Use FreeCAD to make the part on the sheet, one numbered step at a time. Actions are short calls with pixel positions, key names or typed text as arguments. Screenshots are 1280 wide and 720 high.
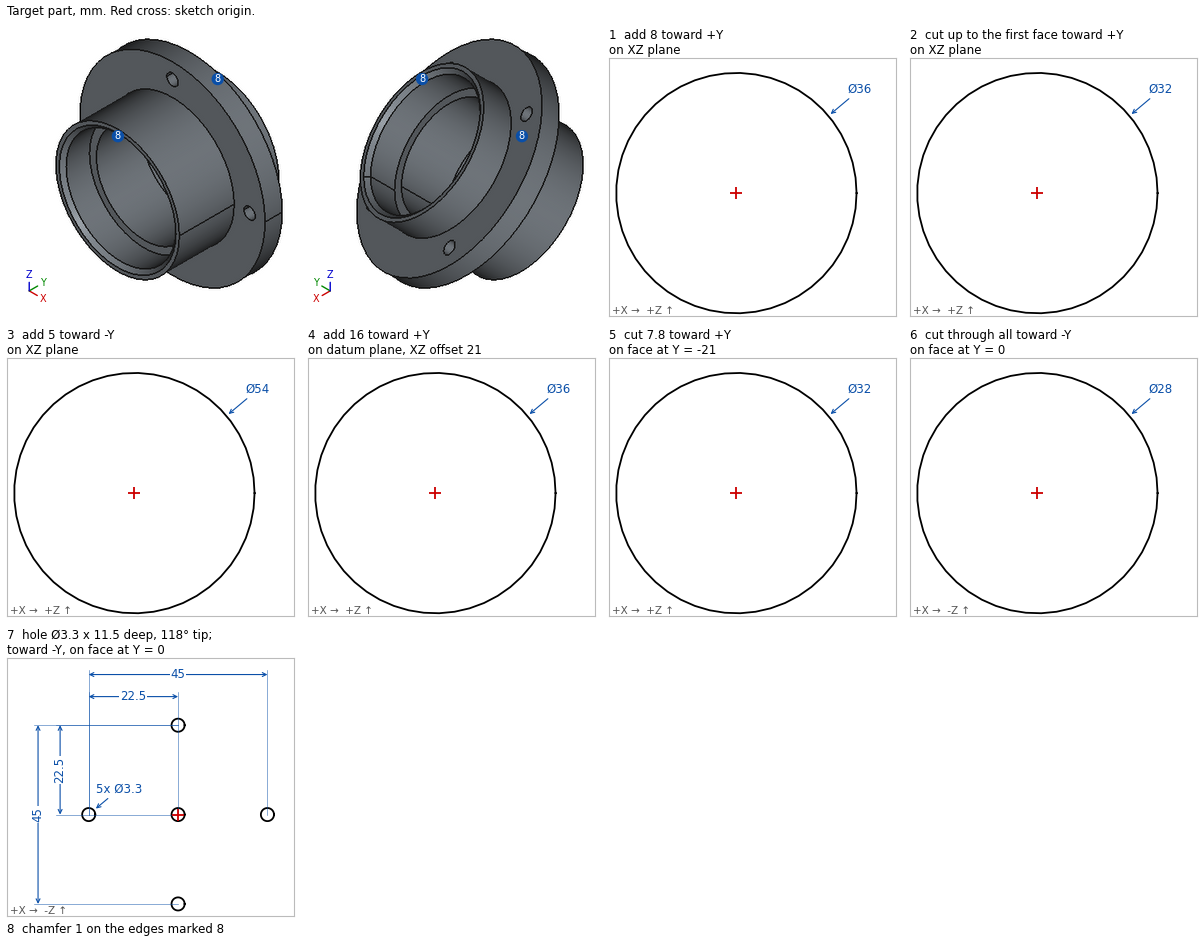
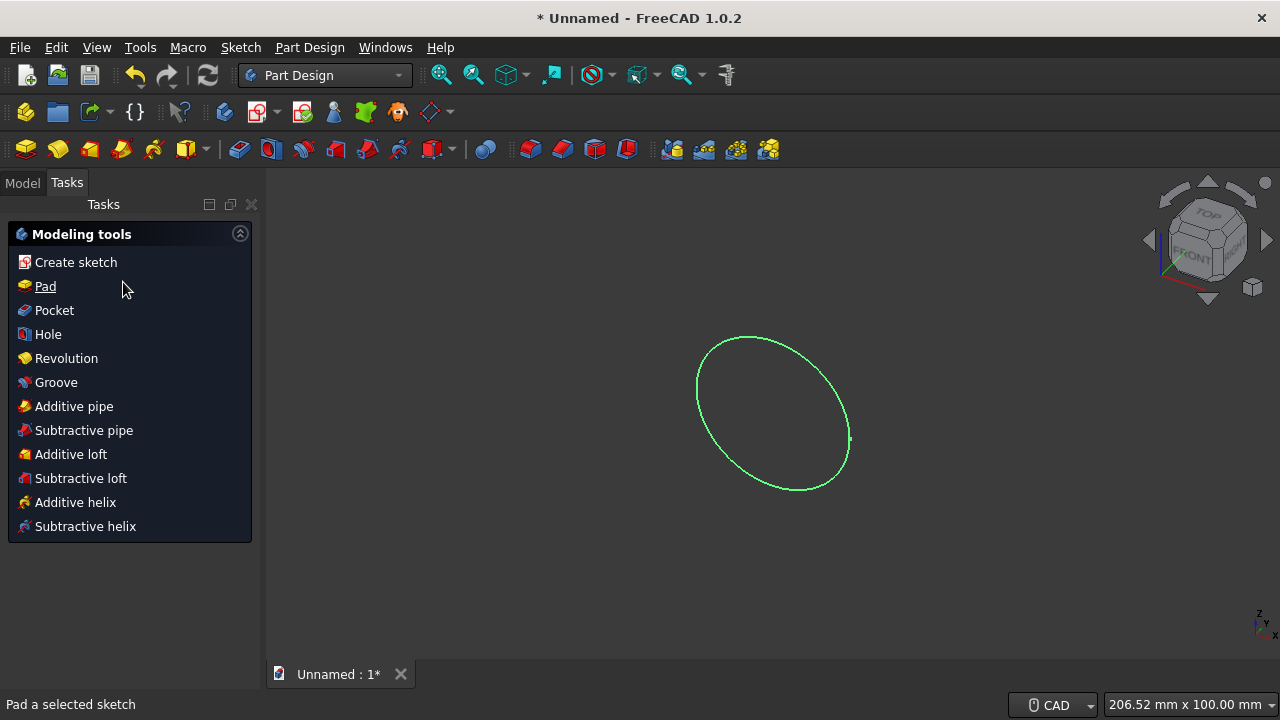
click(26, 150)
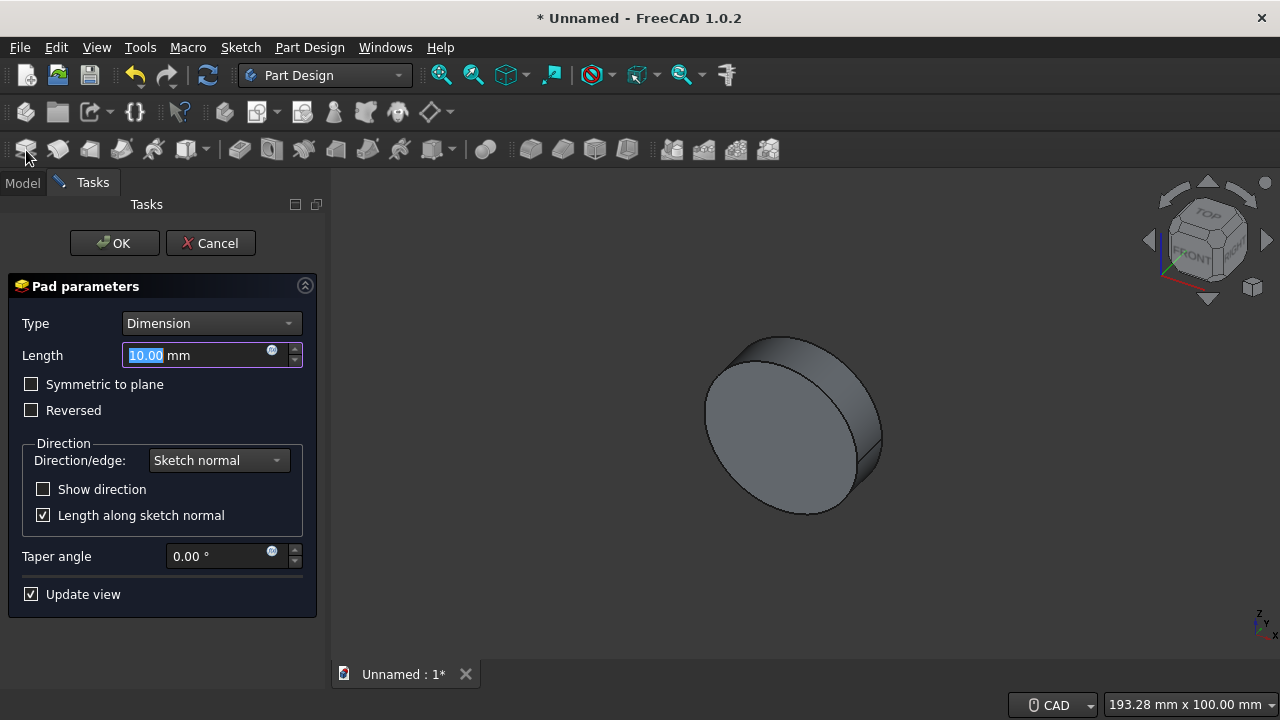
text(8)
key(Tab)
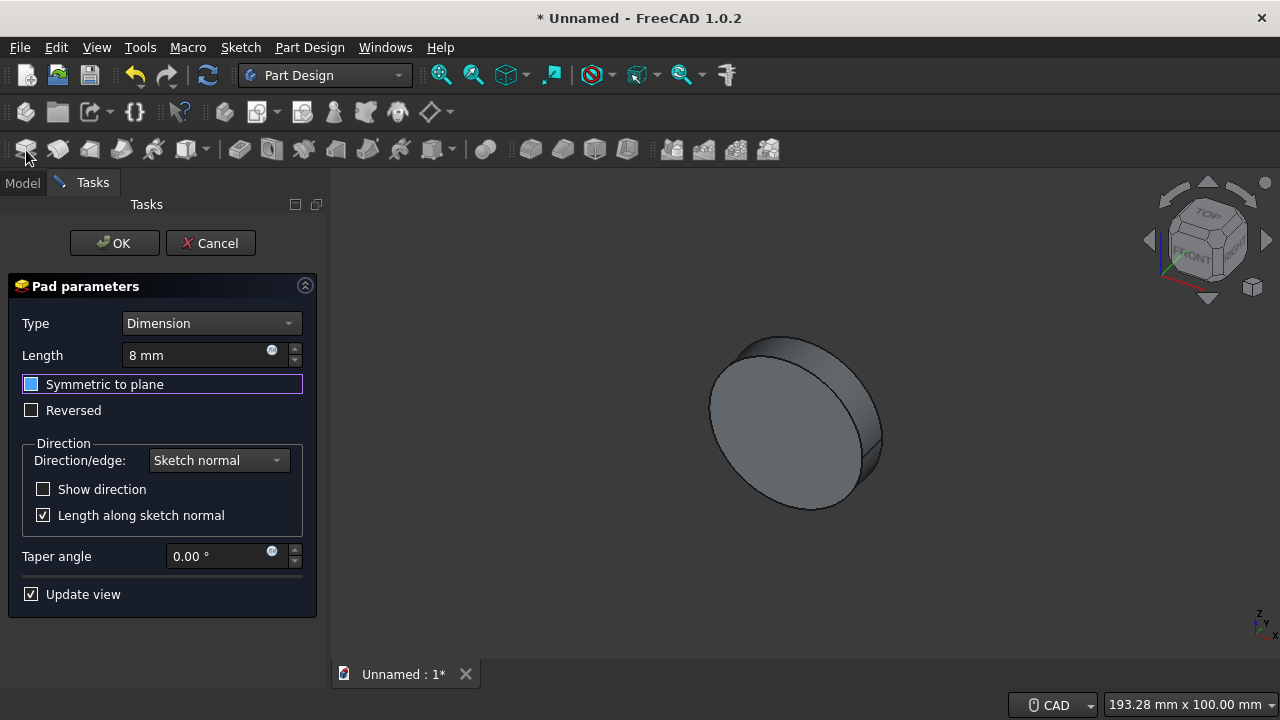
click(30, 410)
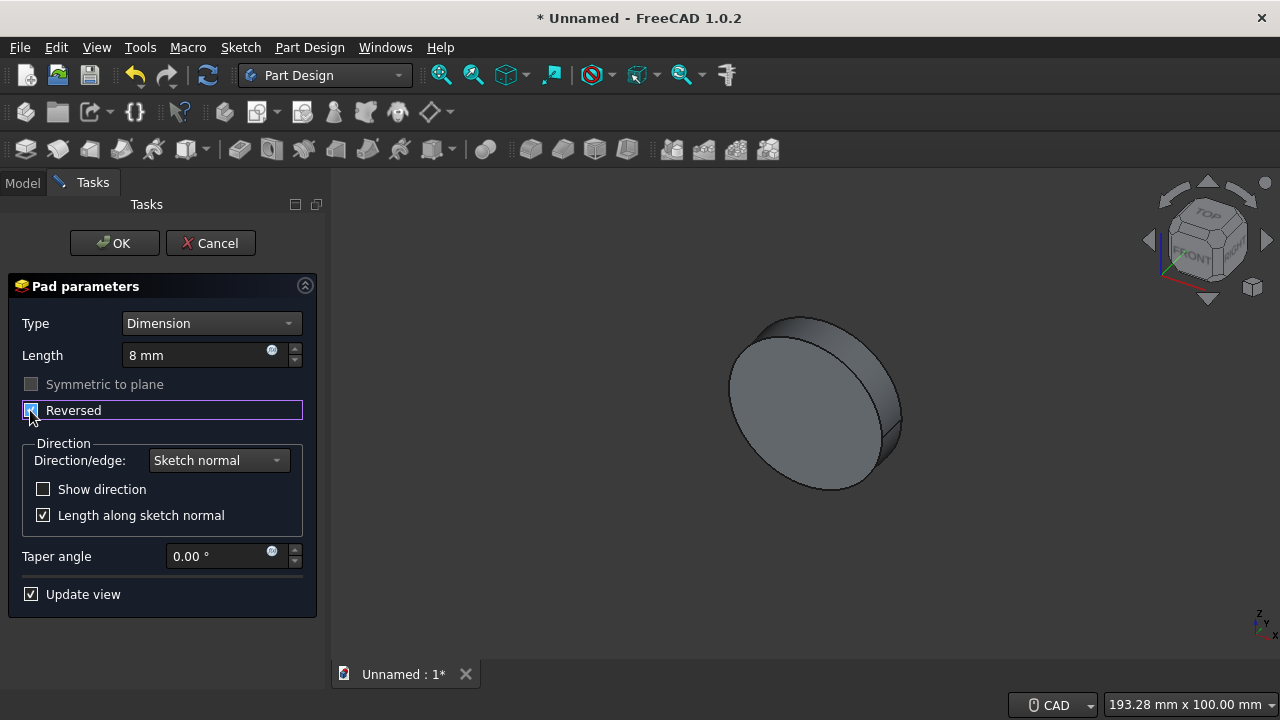
click(115, 243)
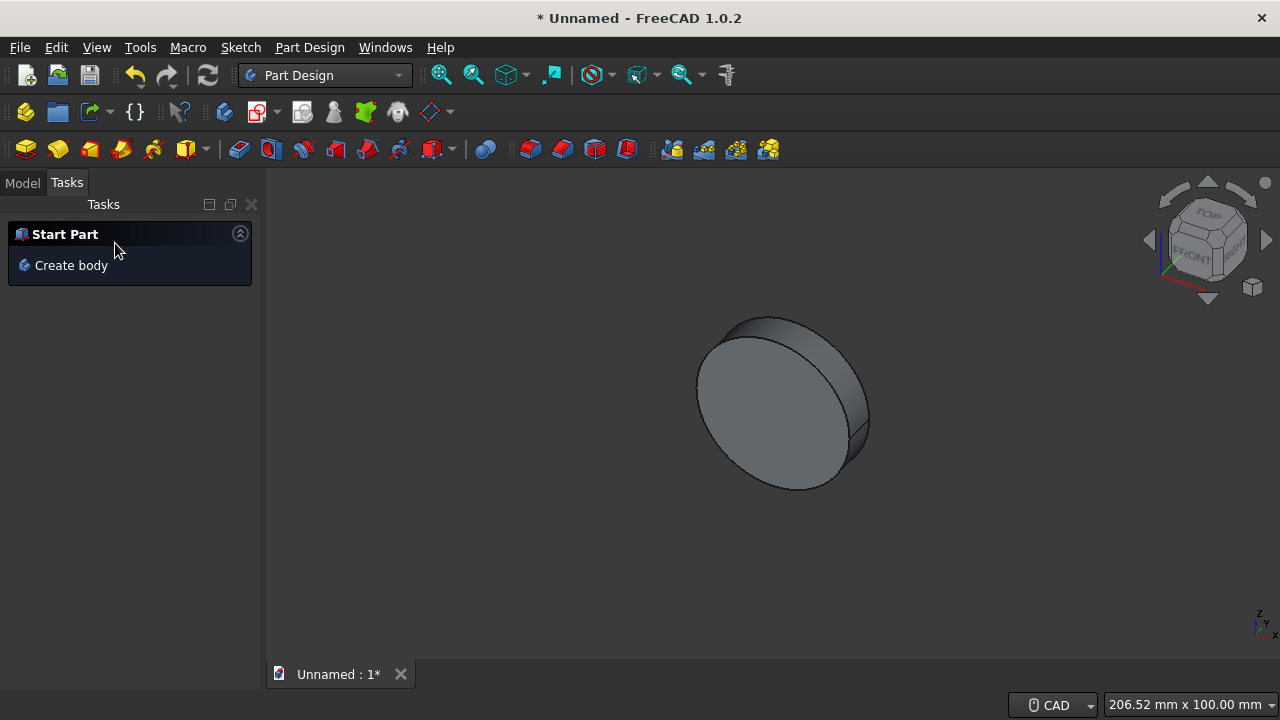
click(442, 76)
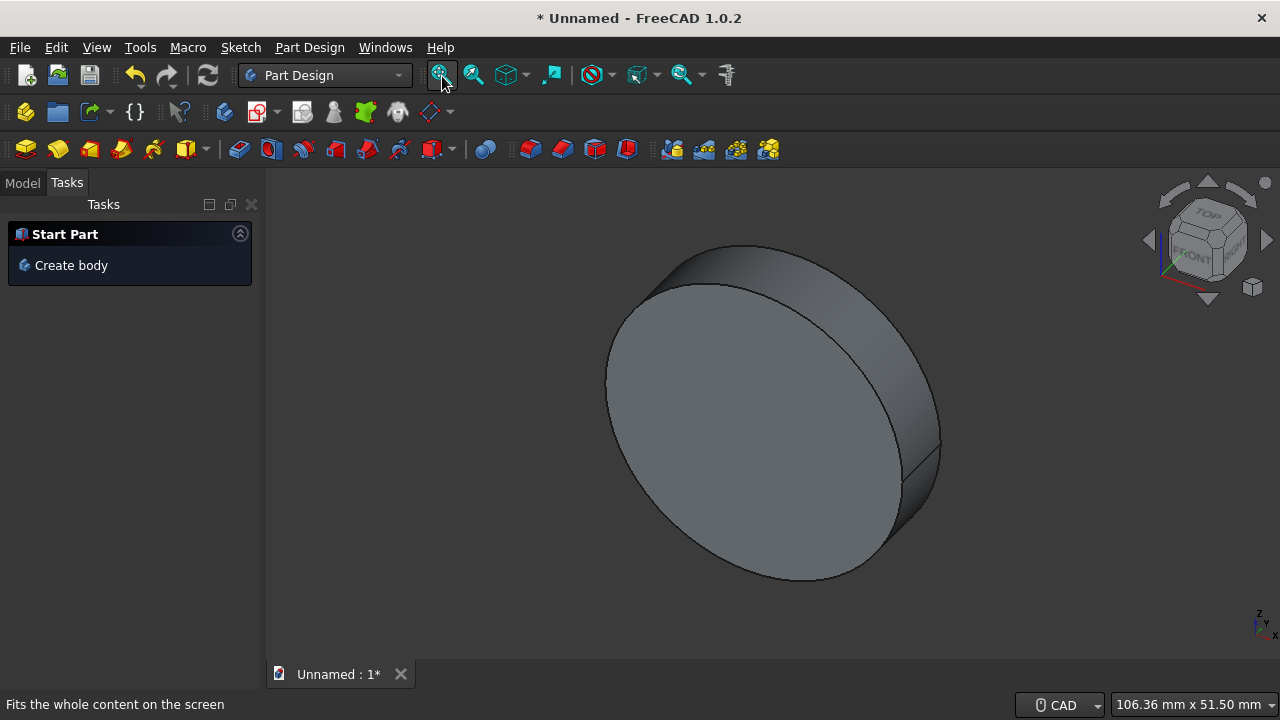
click(258, 112)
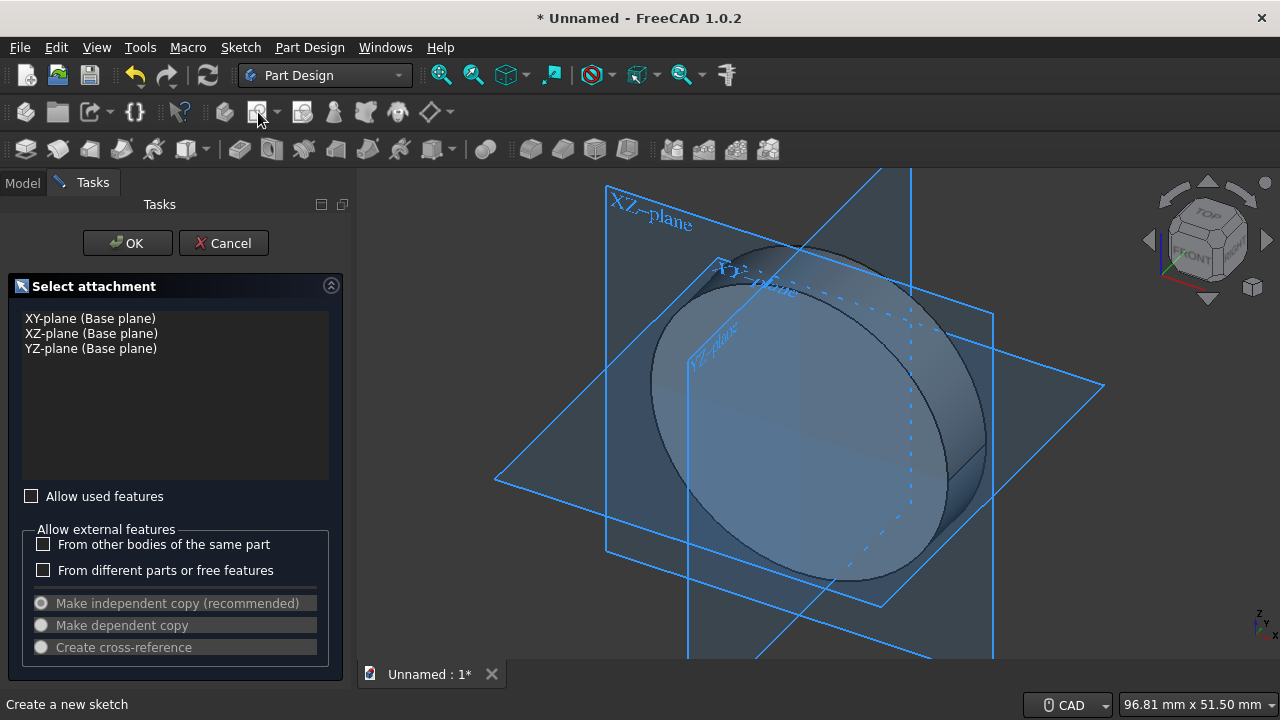
click(82, 334)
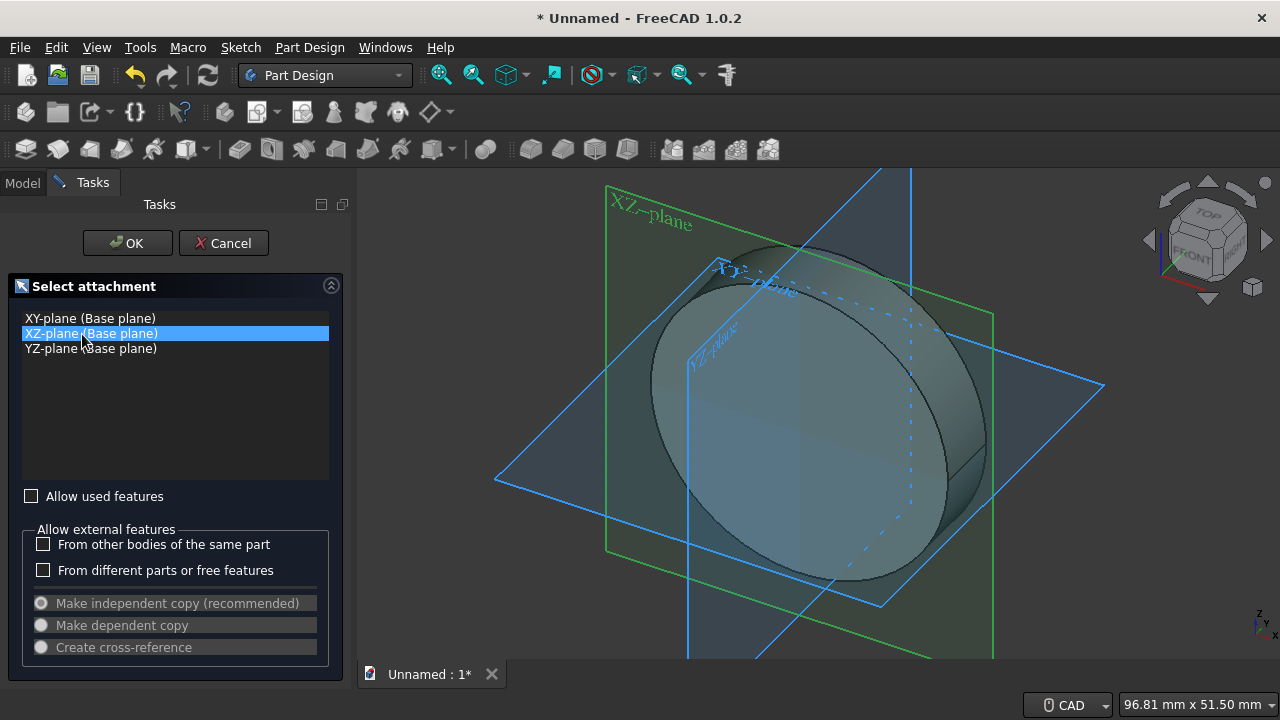
click(128, 243)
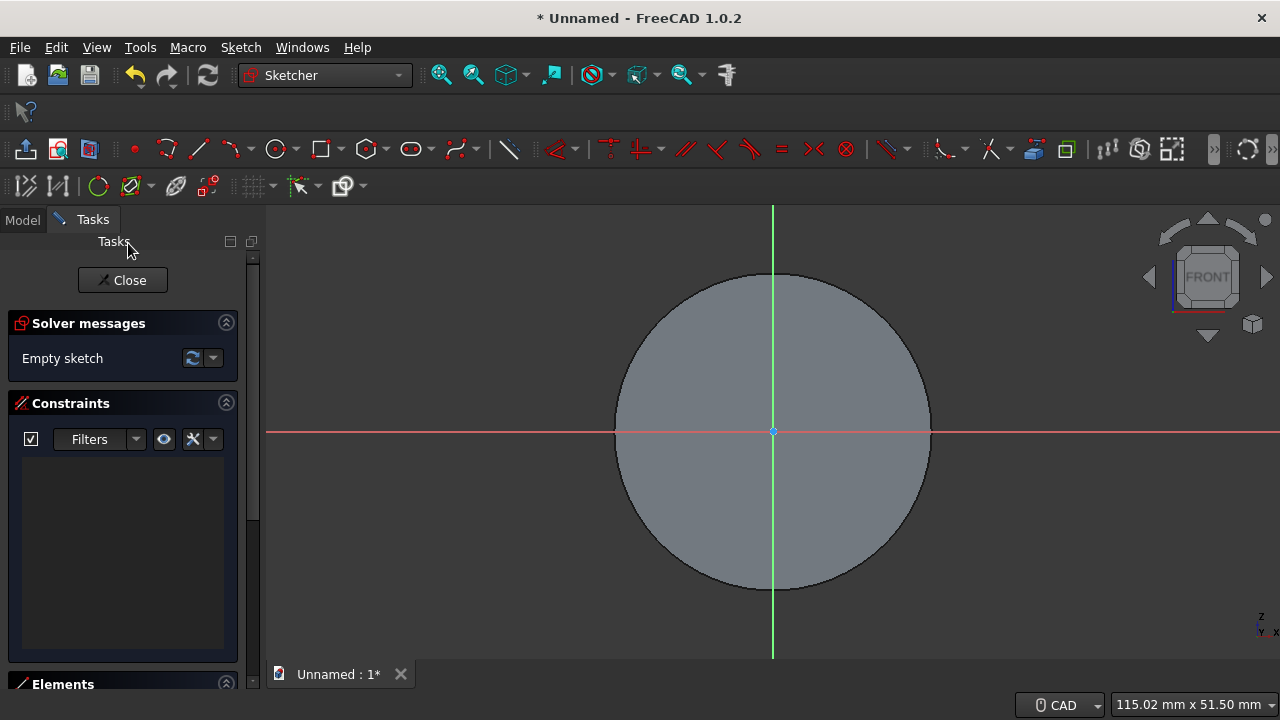
click(276, 150)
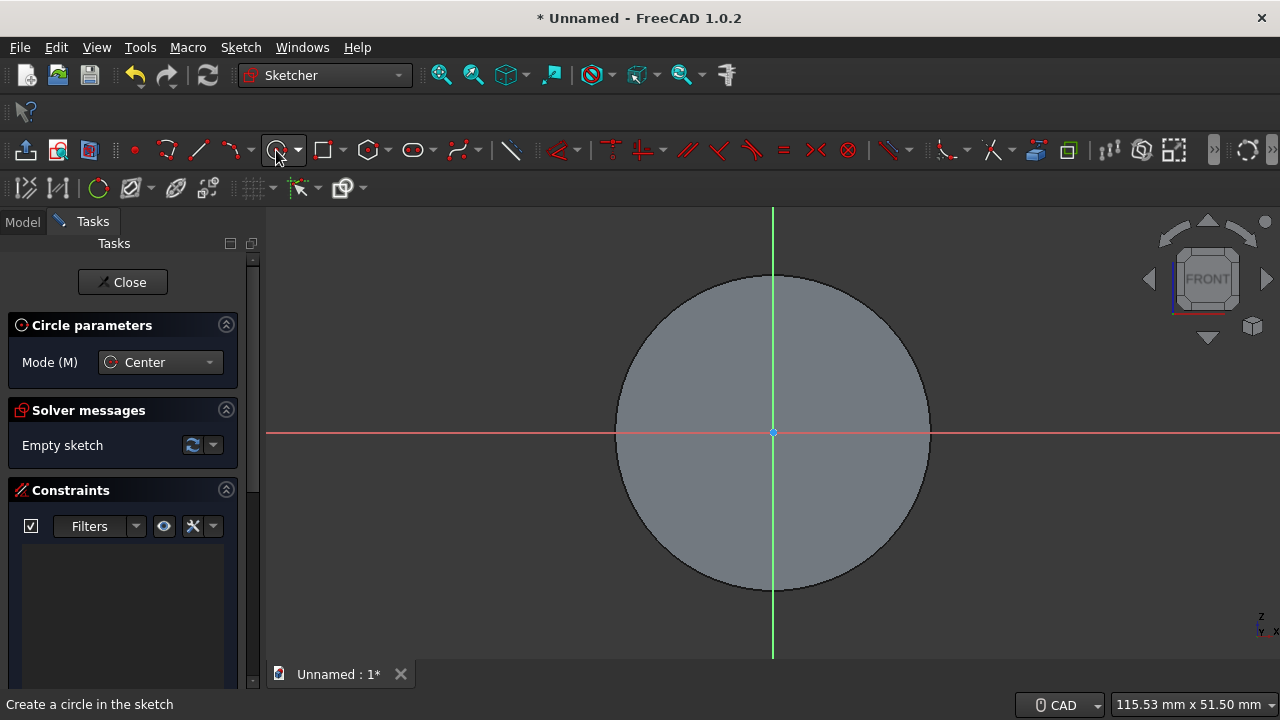
click(773, 433)
click(872, 334)
key(Escape)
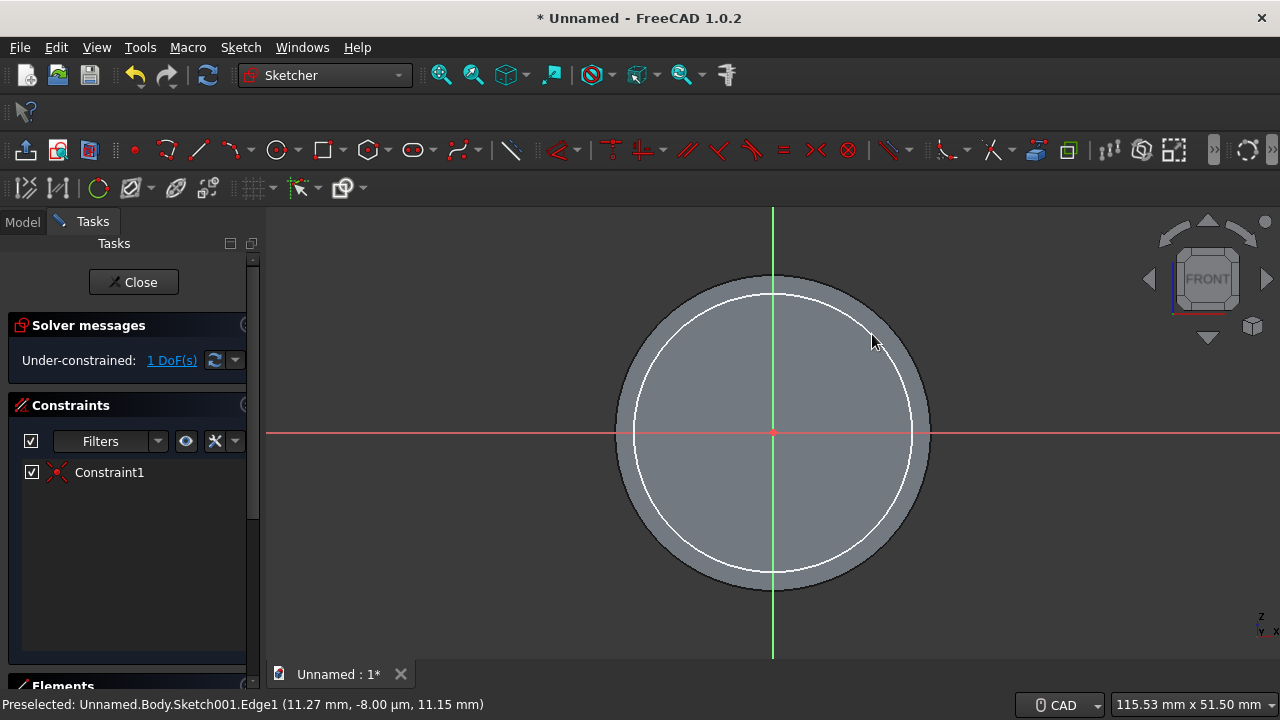
click(871, 334)